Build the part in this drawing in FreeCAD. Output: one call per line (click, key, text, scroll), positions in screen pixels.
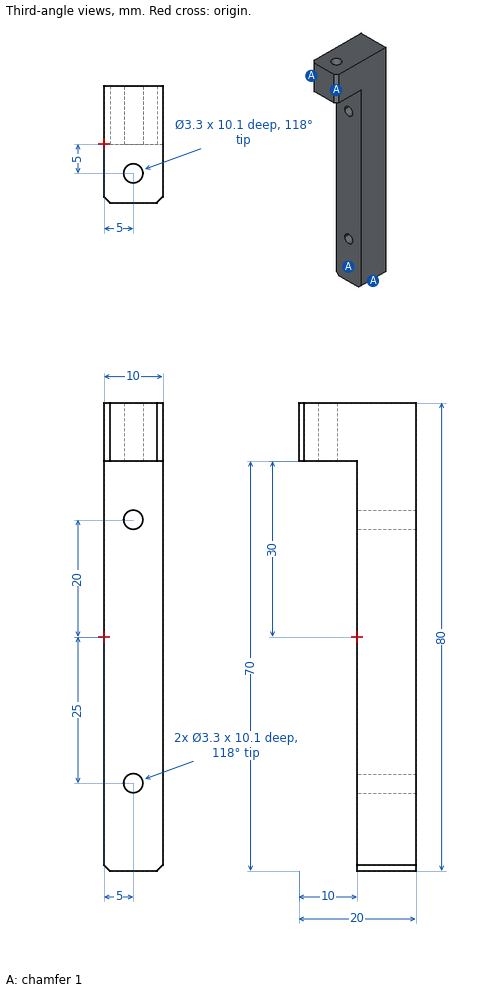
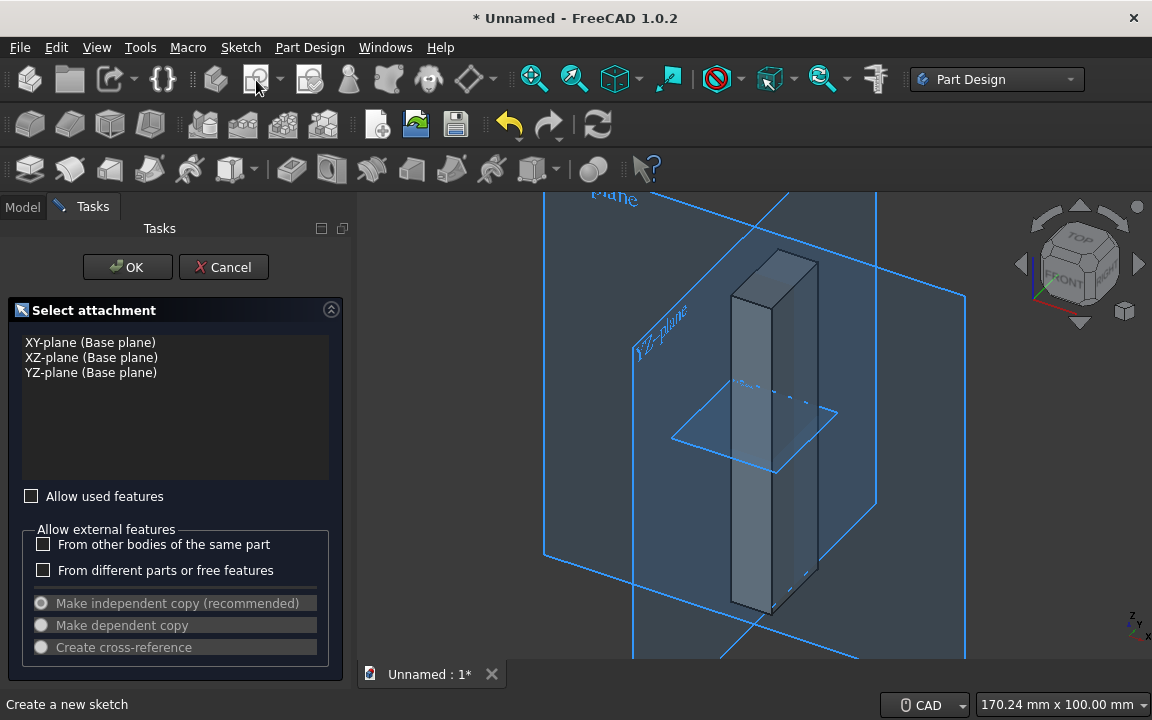
click(82, 372)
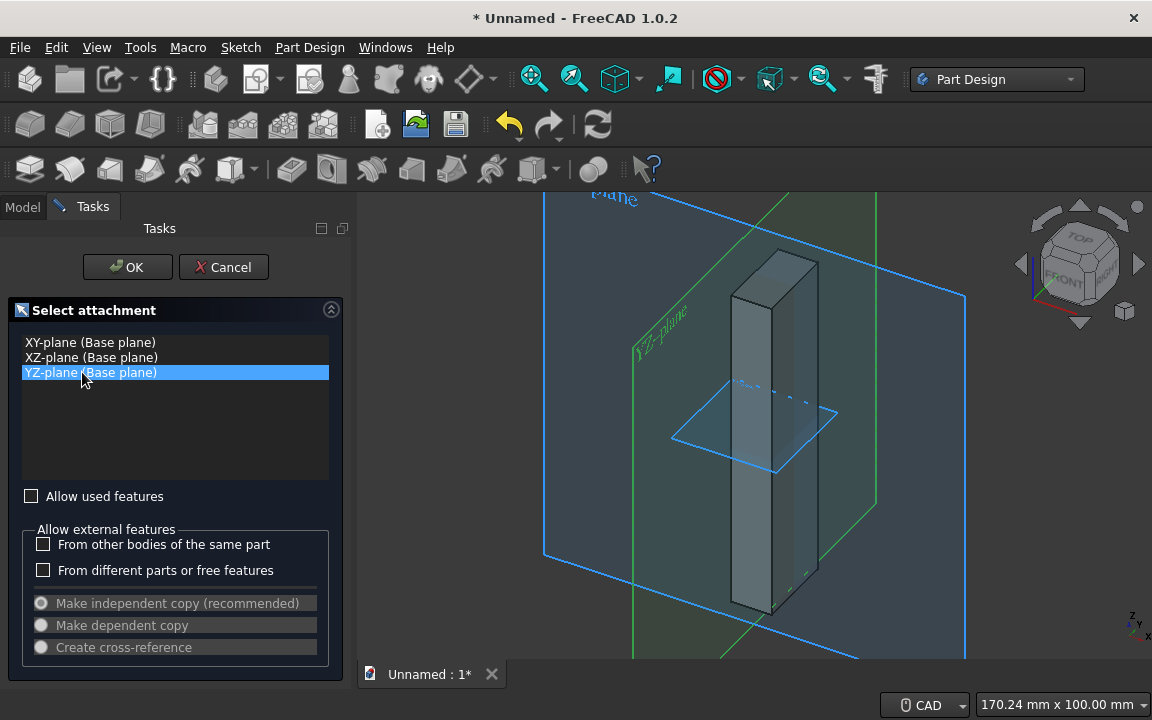
click(128, 267)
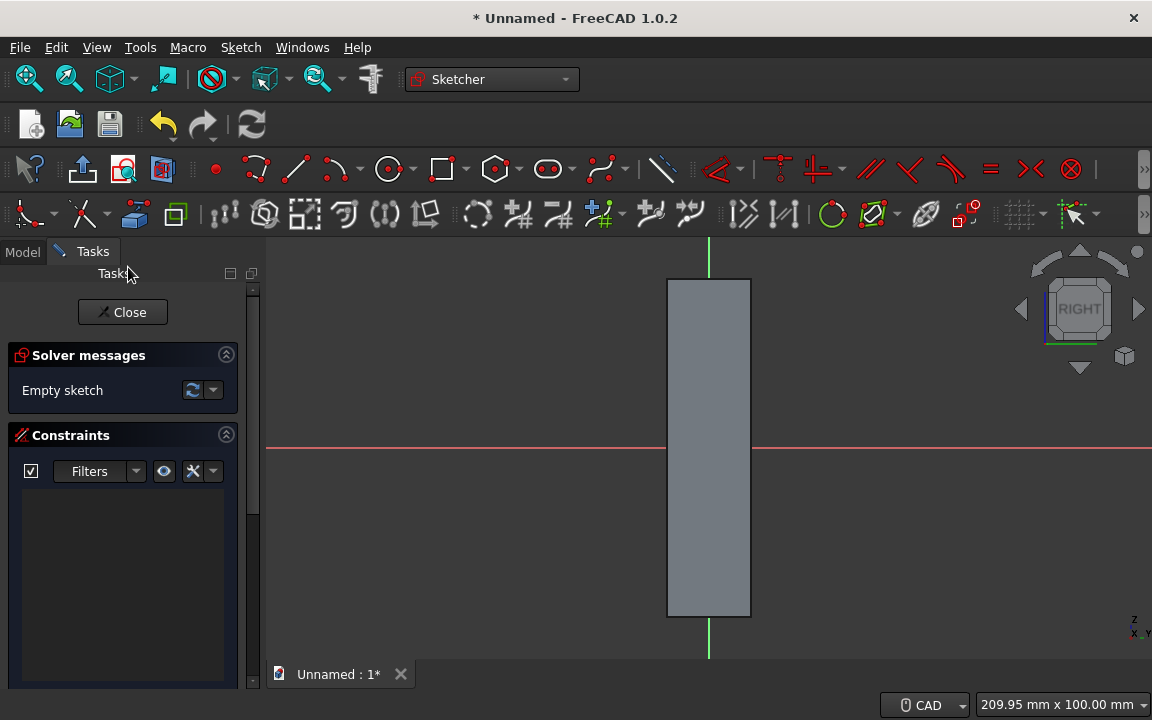
click(164, 170)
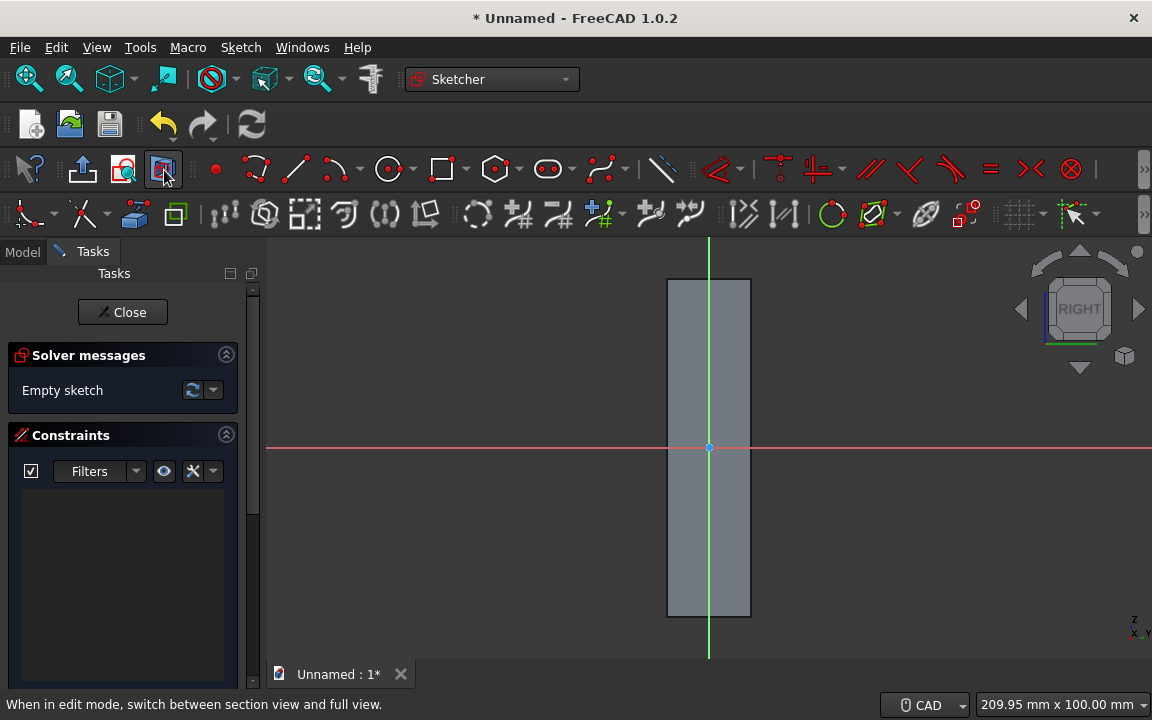
scroll(426, 353, down, 1)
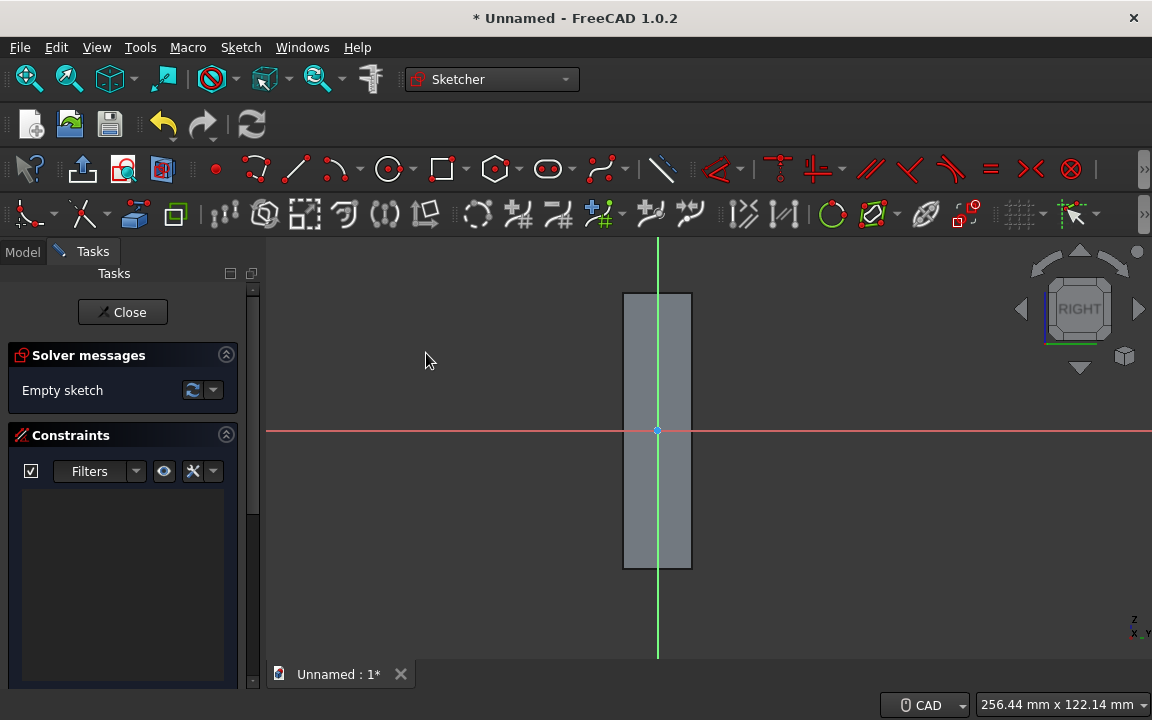
key(g)
key(r)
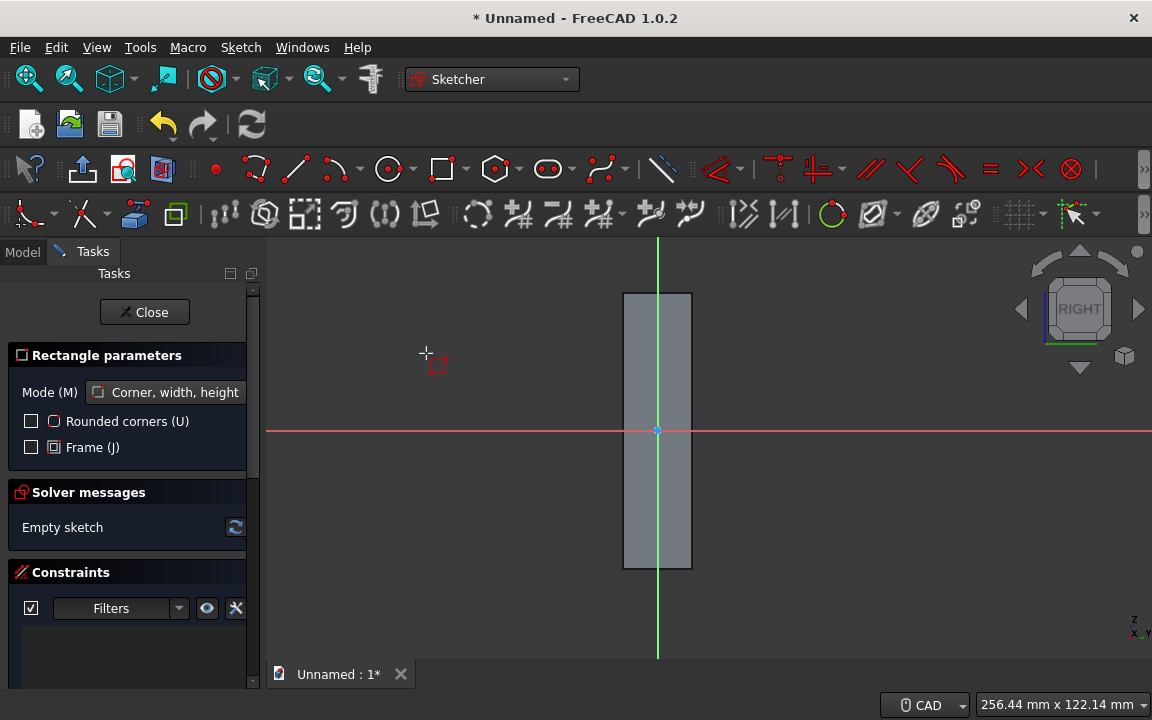
click(623, 327)
click(658, 569)
key(Escape)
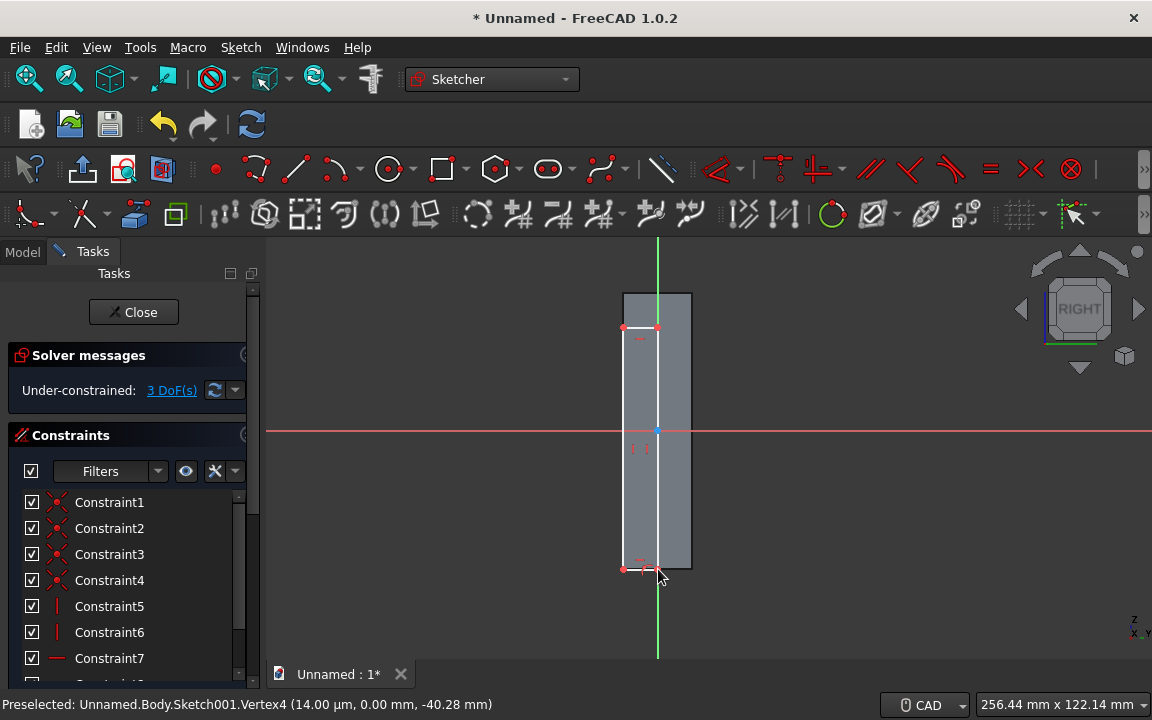
click(623, 401)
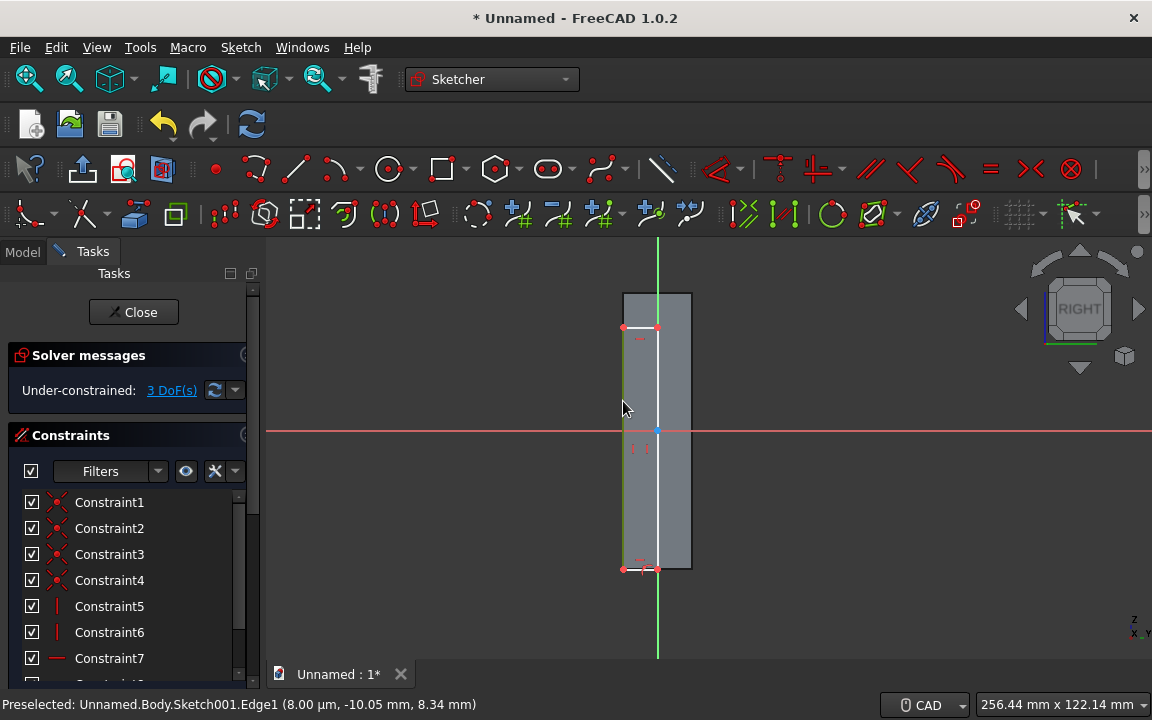
key(i)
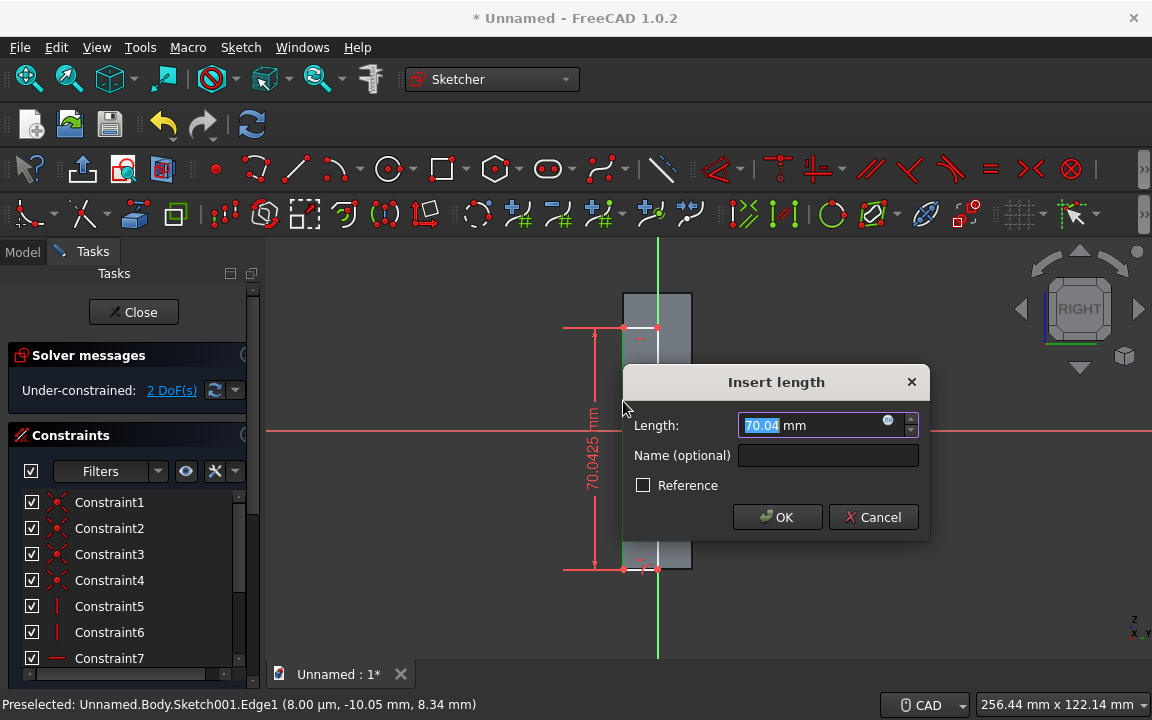
text(70)
key(Return)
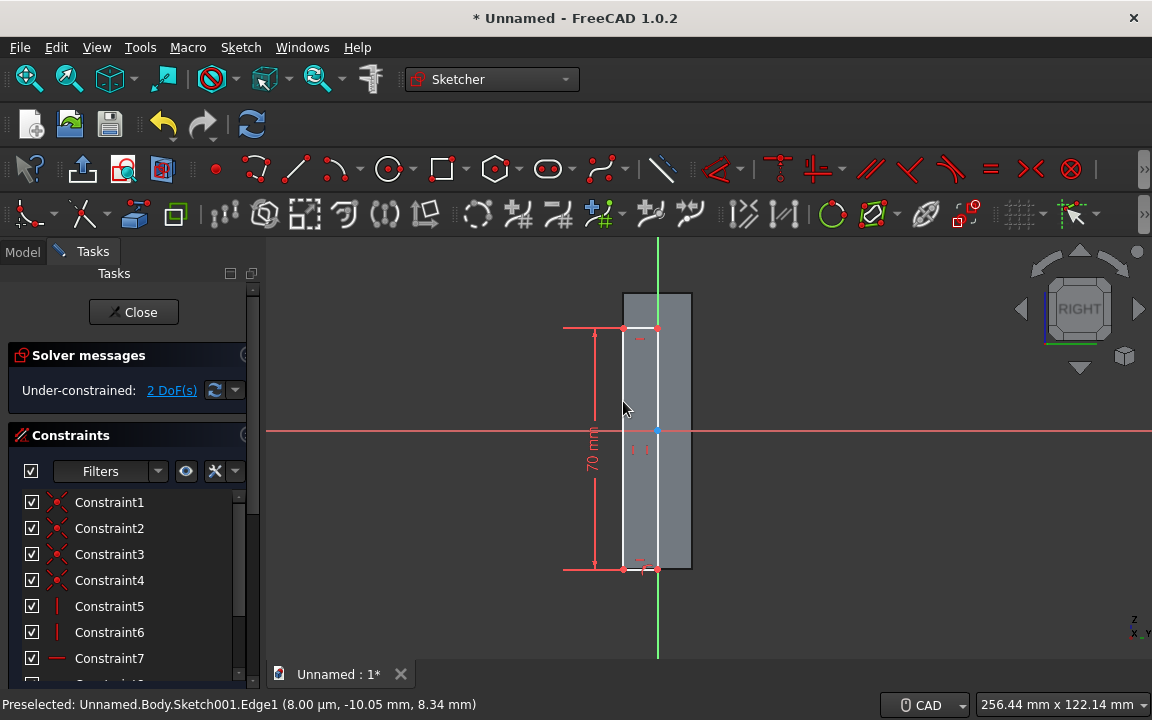
scroll(633, 570, up, 2)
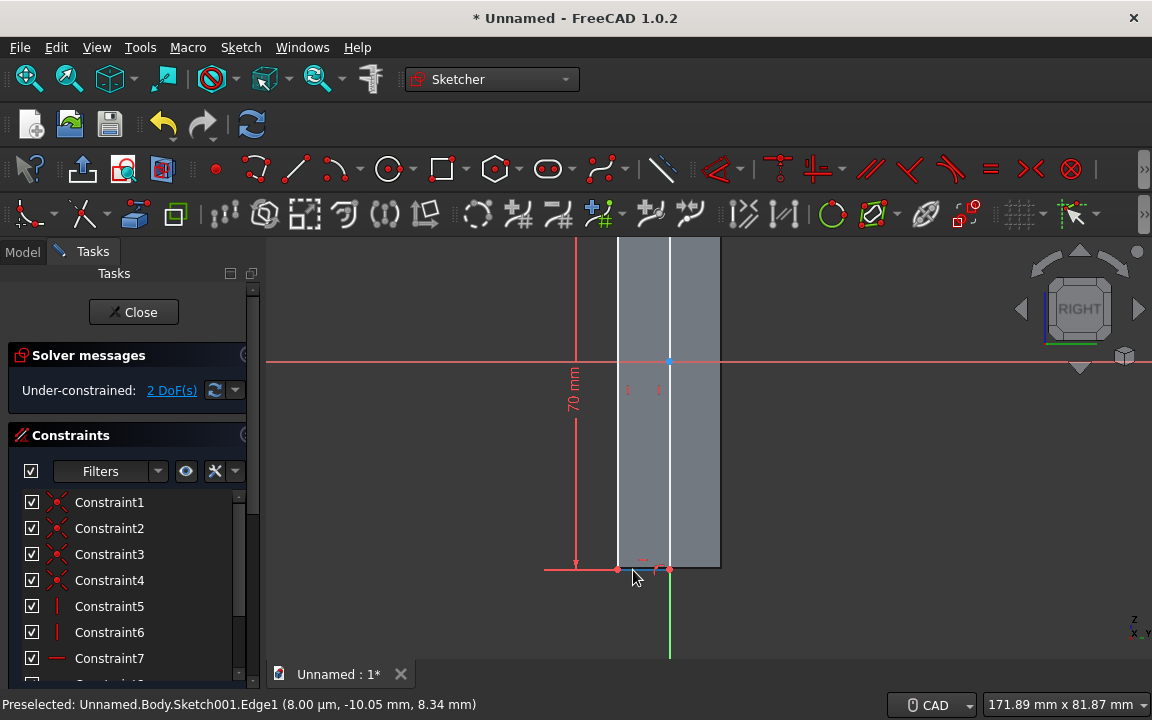
click(633, 570)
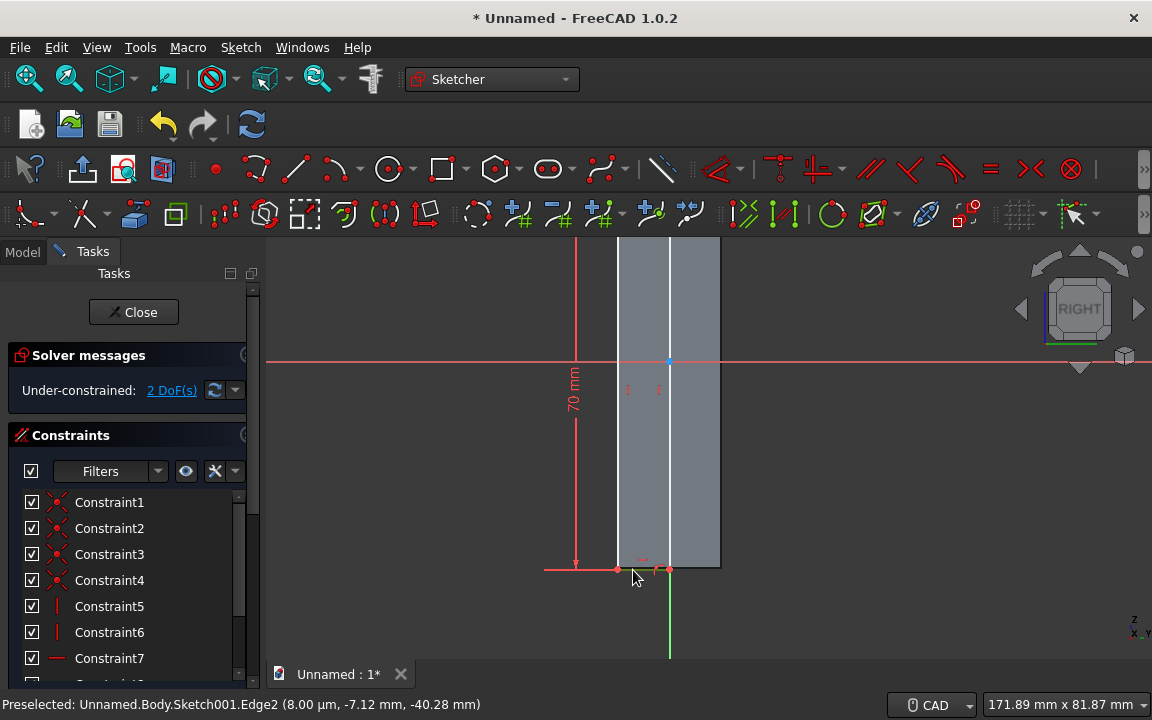
key(l)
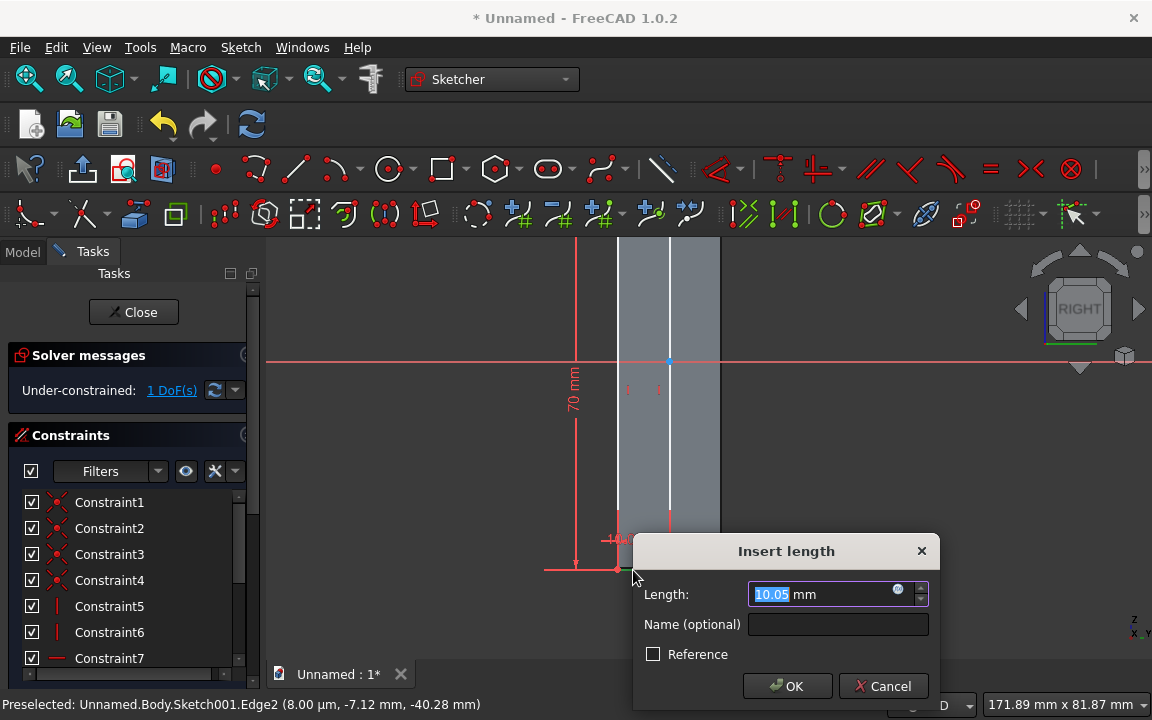
text(10)
key(Return)